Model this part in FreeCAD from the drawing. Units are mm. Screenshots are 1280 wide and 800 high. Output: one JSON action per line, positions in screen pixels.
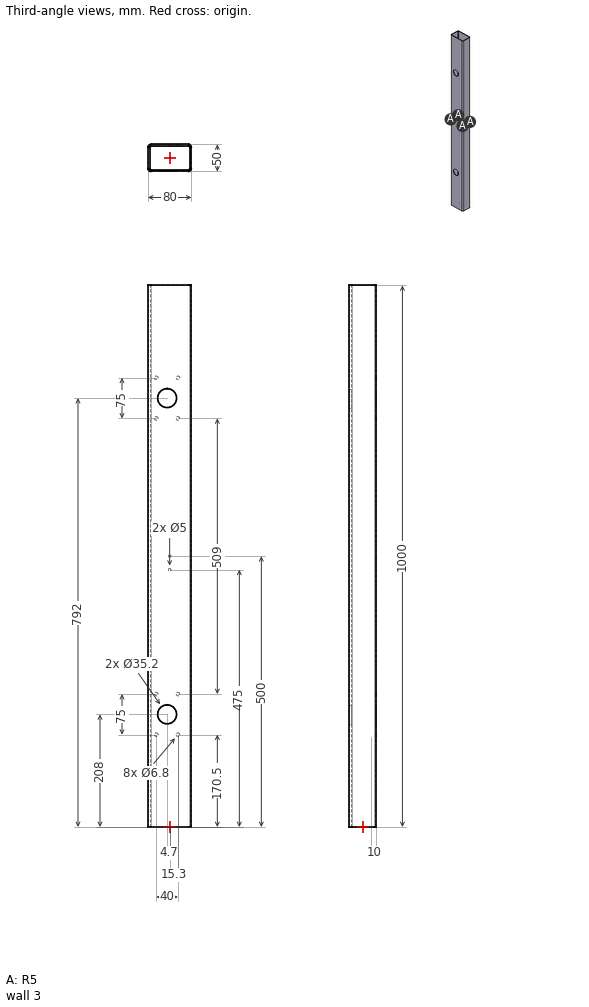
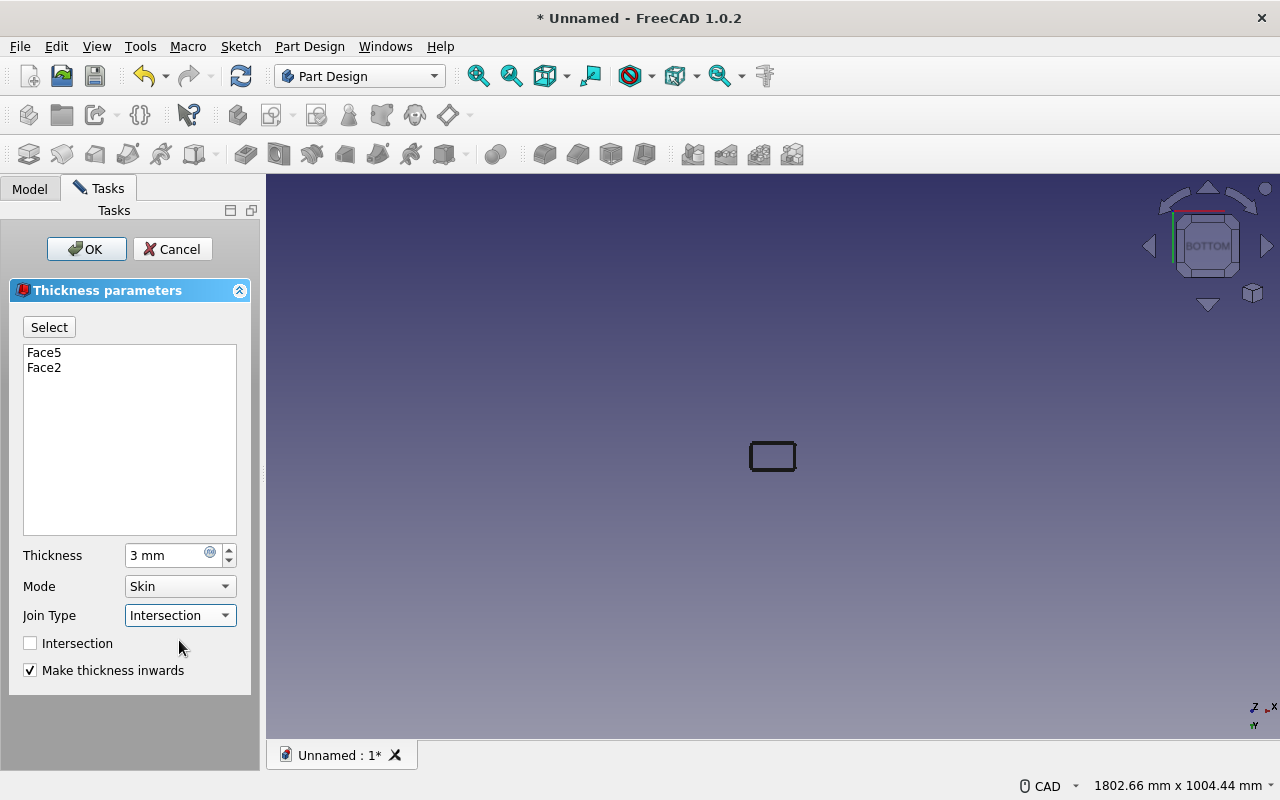
{"action": "left_click", "coordinate": [87, 249]}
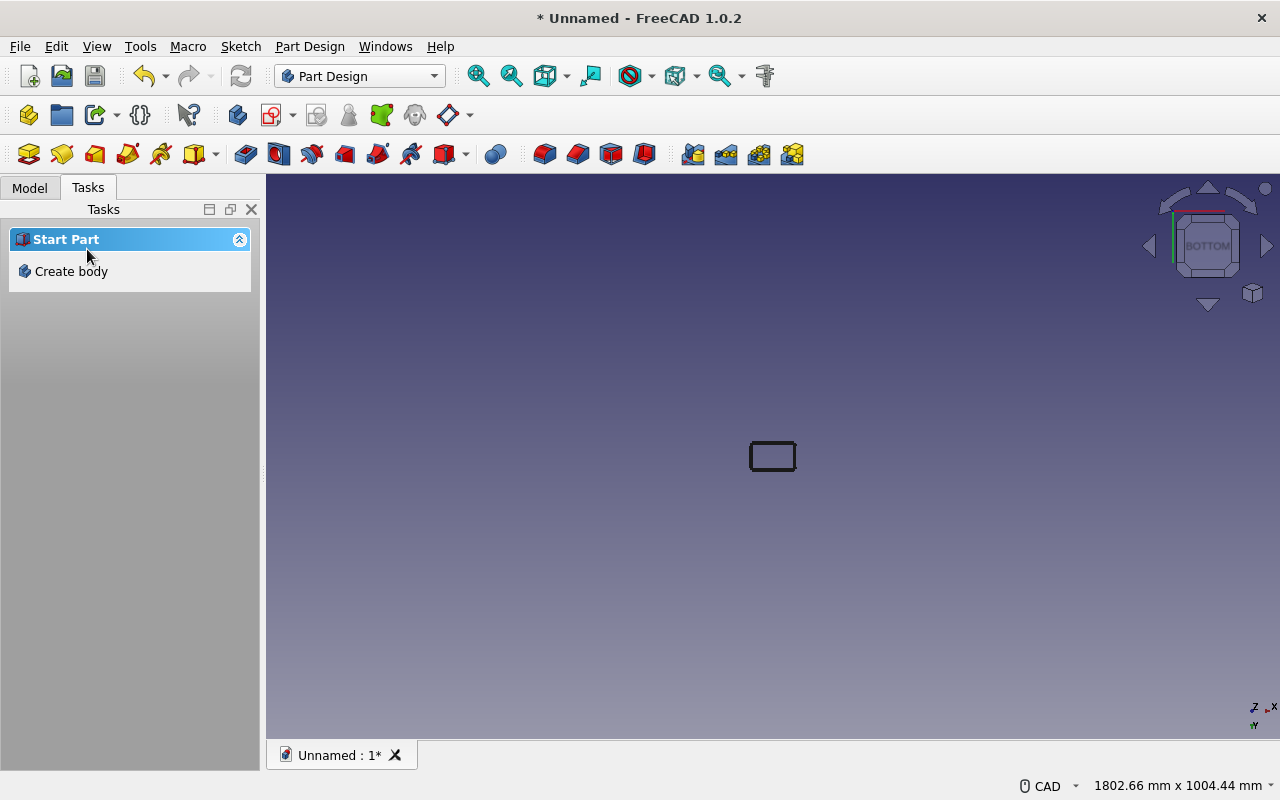
{"action": "left_click", "coordinate": [479, 76]}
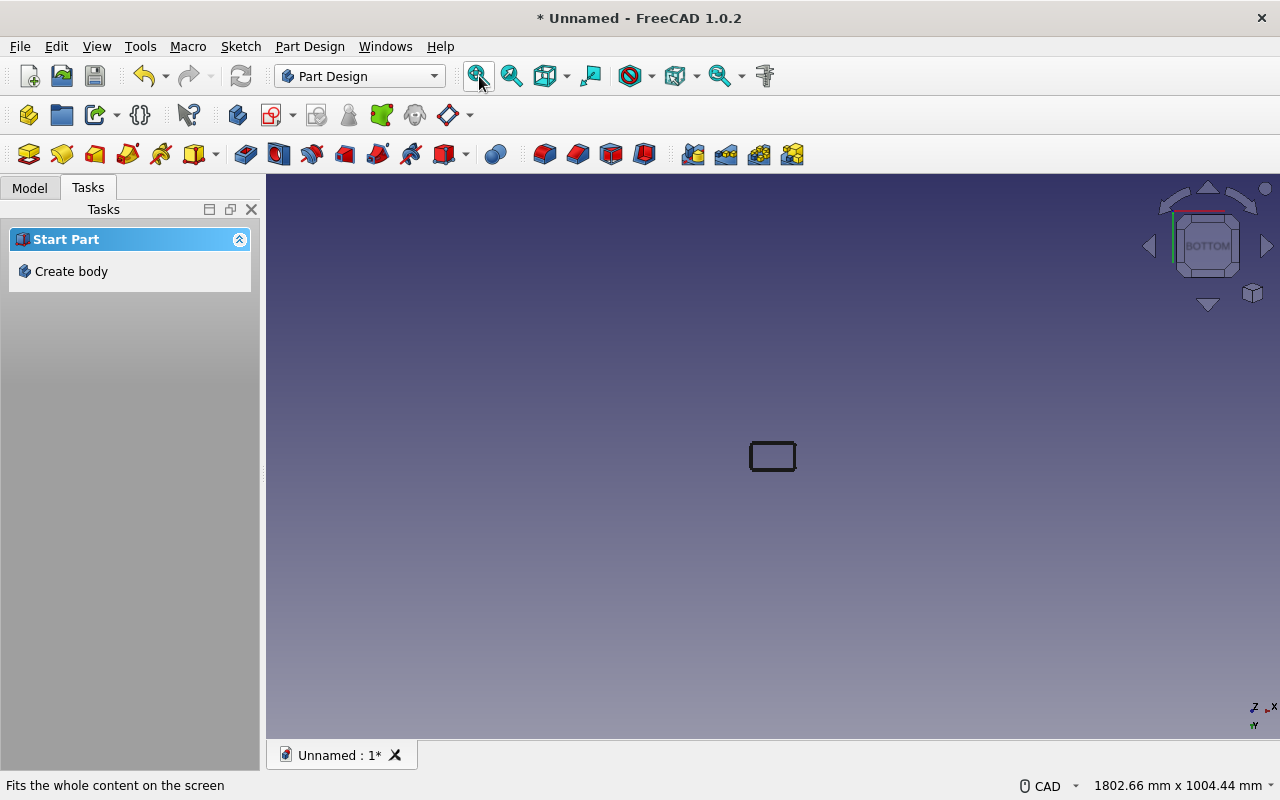
{"action": "key", "text": "4"}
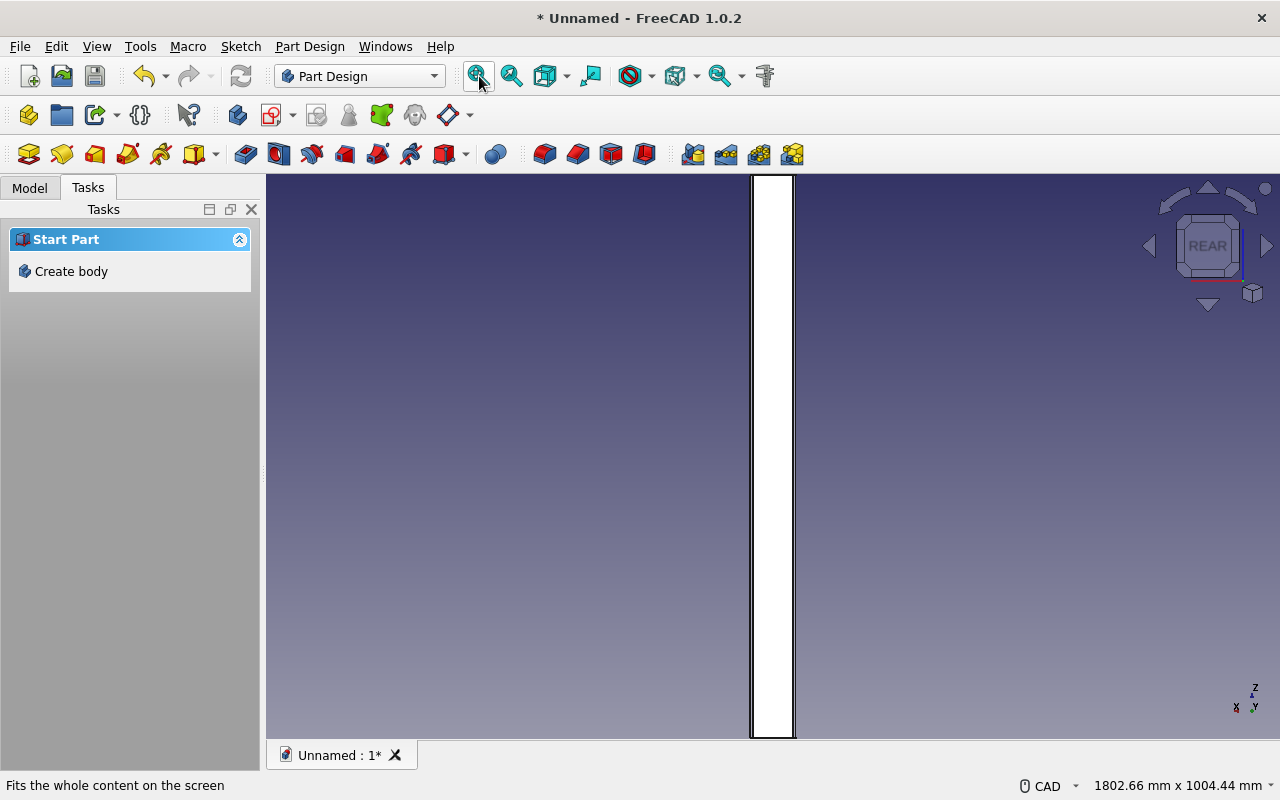
{"action": "left_click", "coordinate": [773, 214]}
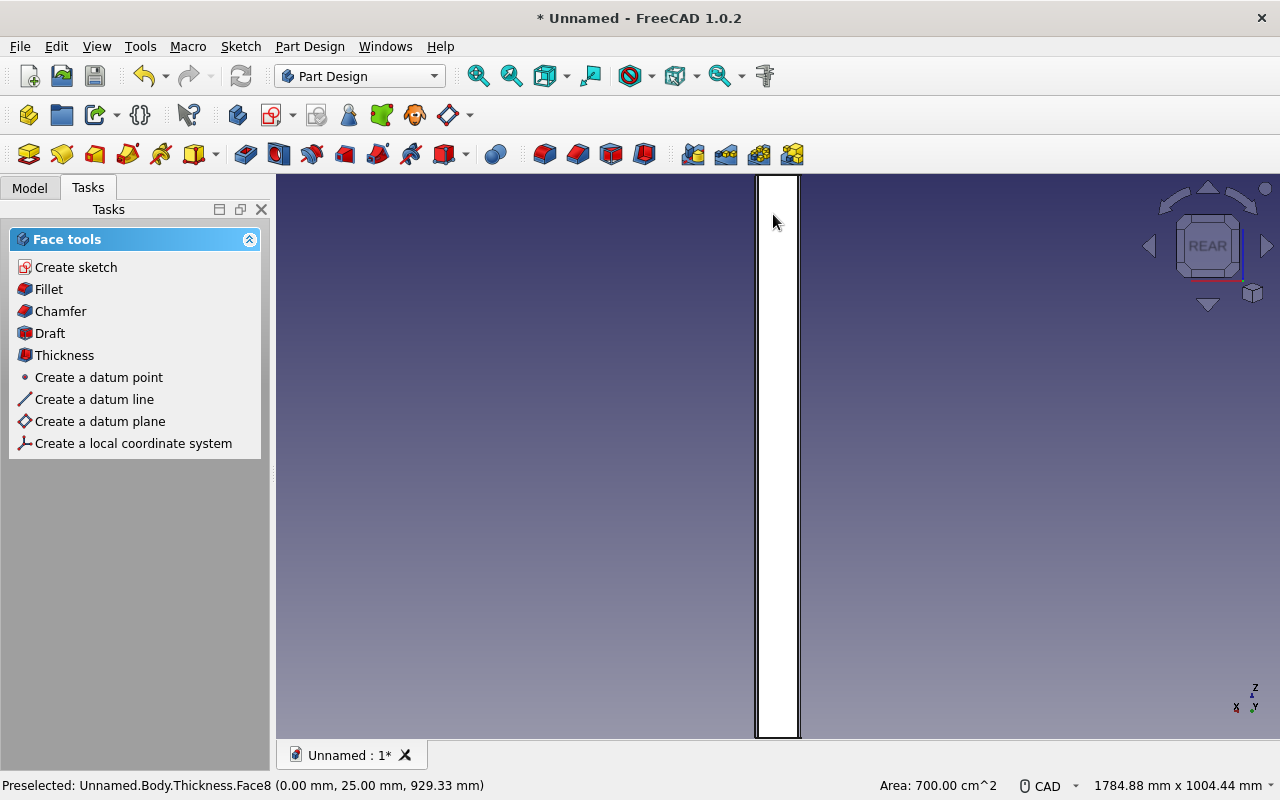
{"action": "left_click", "coordinate": [270, 116]}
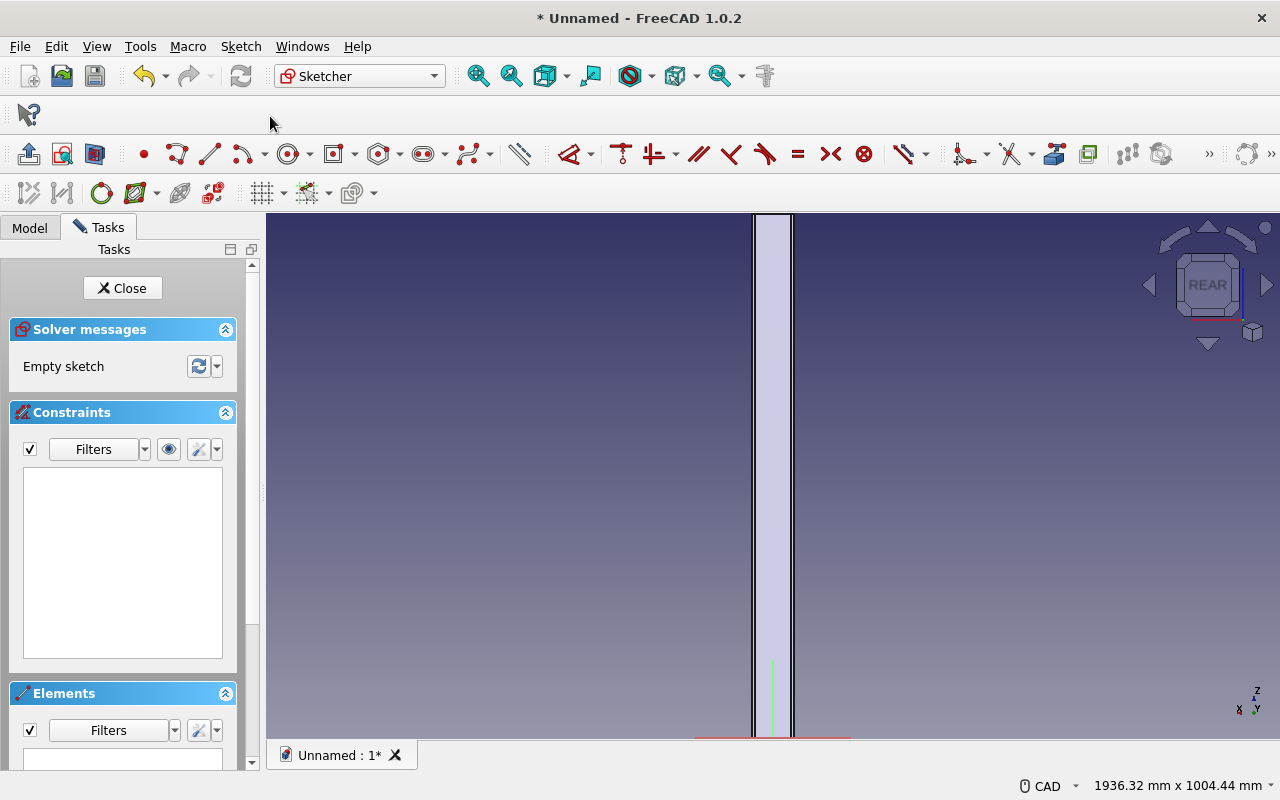
{"action": "scroll", "coordinate": [384, 251], "scroll_direction": "down", "scroll_amount": 1}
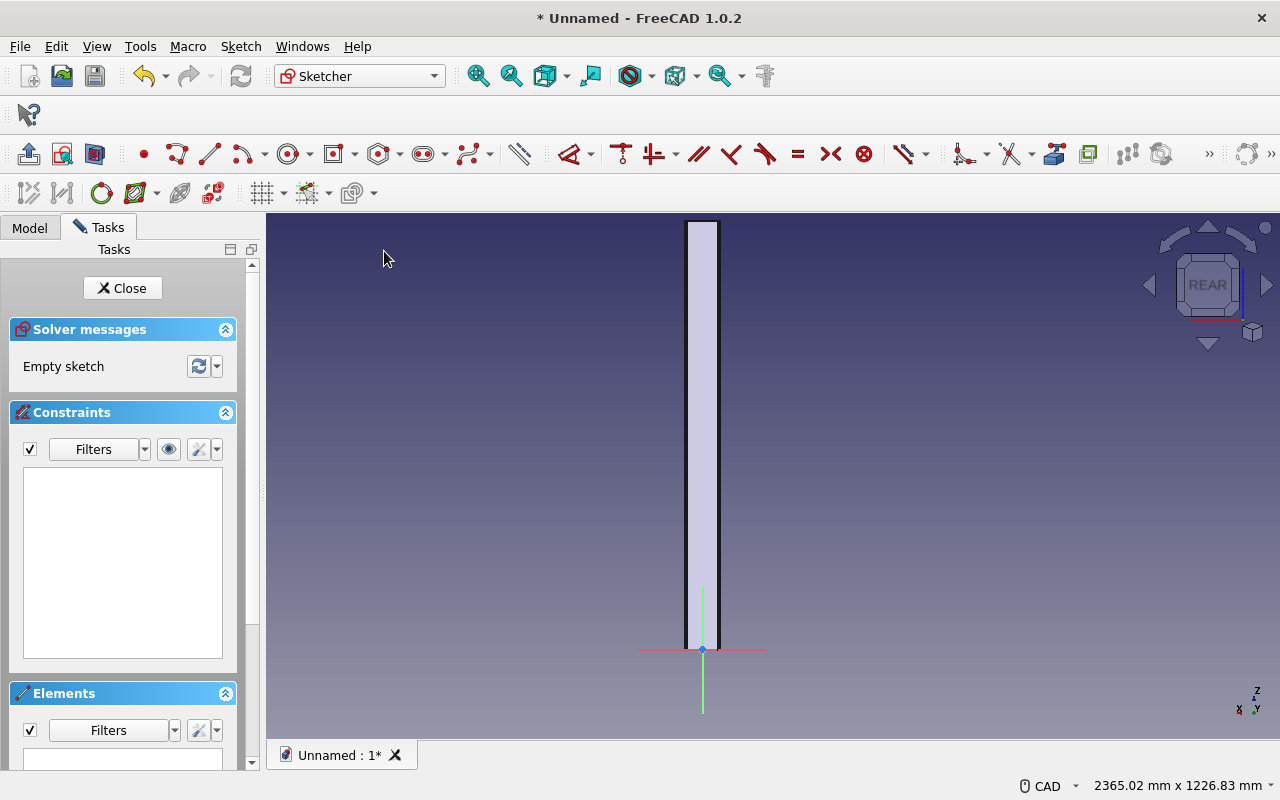
{"action": "left_click", "coordinate": [288, 154]}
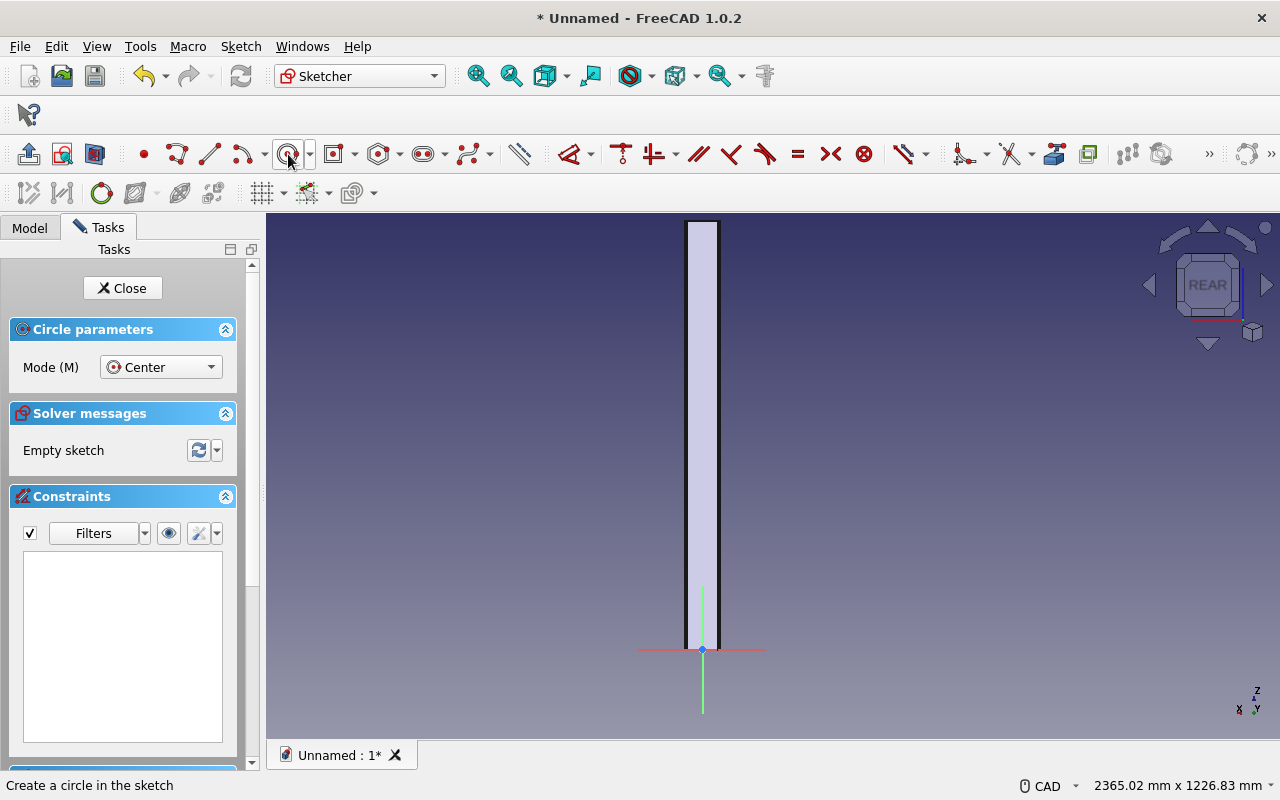
{"action": "scroll", "coordinate": [705, 560], "scroll_direction": "up", "scroll_amount": 11}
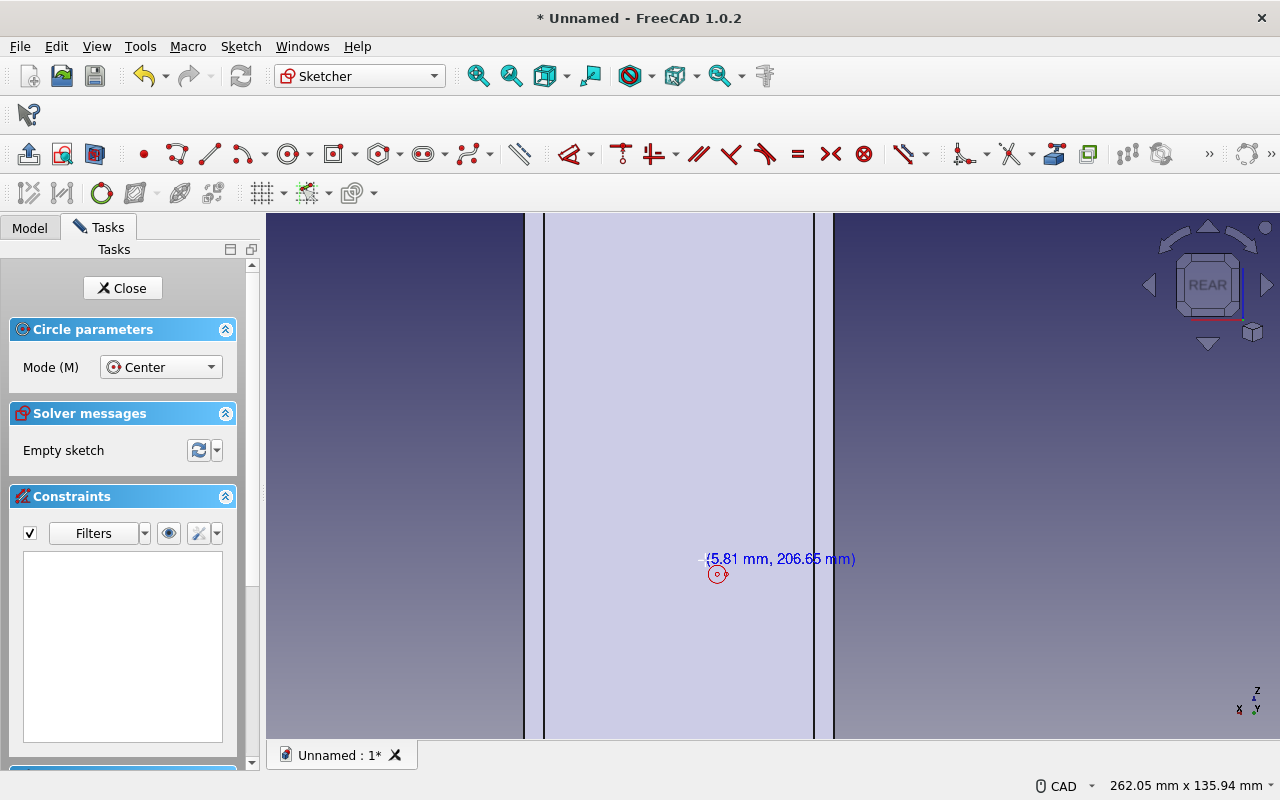
{"action": "left_click", "coordinate": [697, 559]}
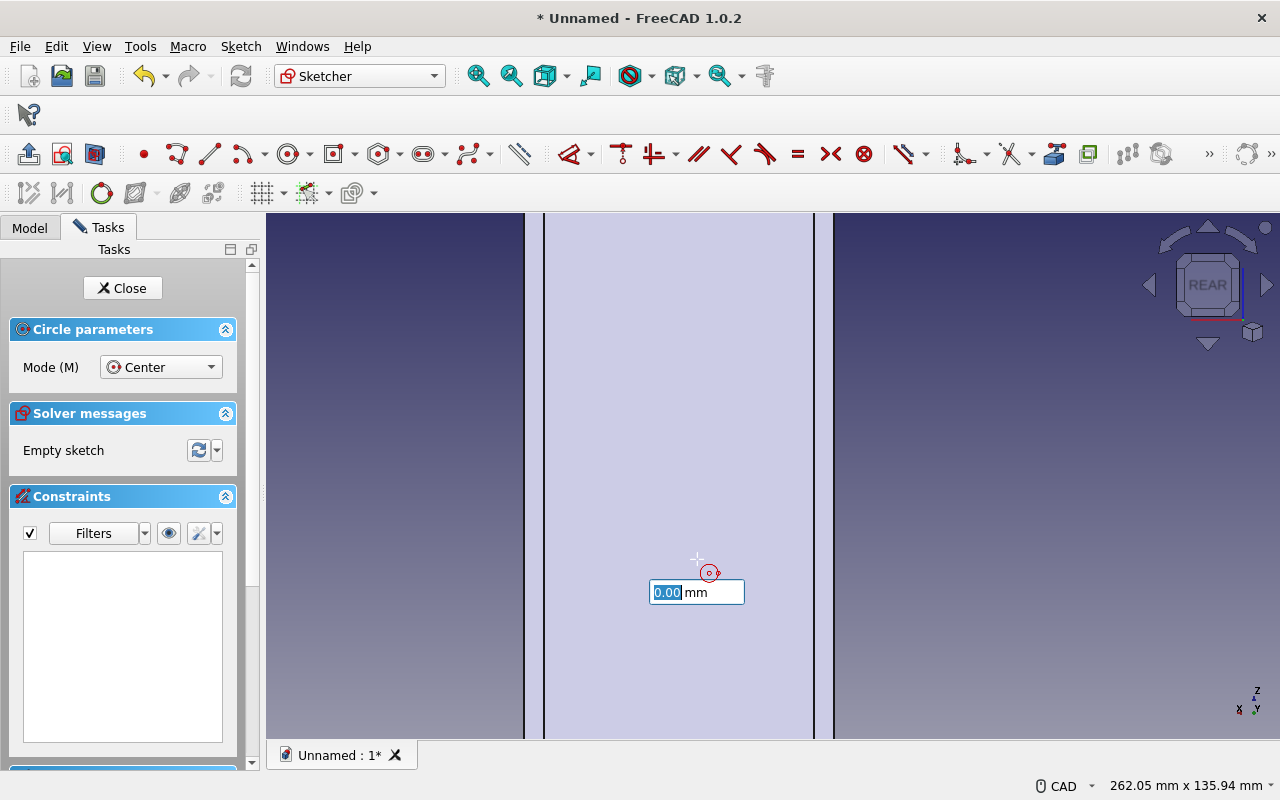
{"action": "scroll", "coordinate": [705, 561], "scroll_direction": "down", "scroll_amount": 11}